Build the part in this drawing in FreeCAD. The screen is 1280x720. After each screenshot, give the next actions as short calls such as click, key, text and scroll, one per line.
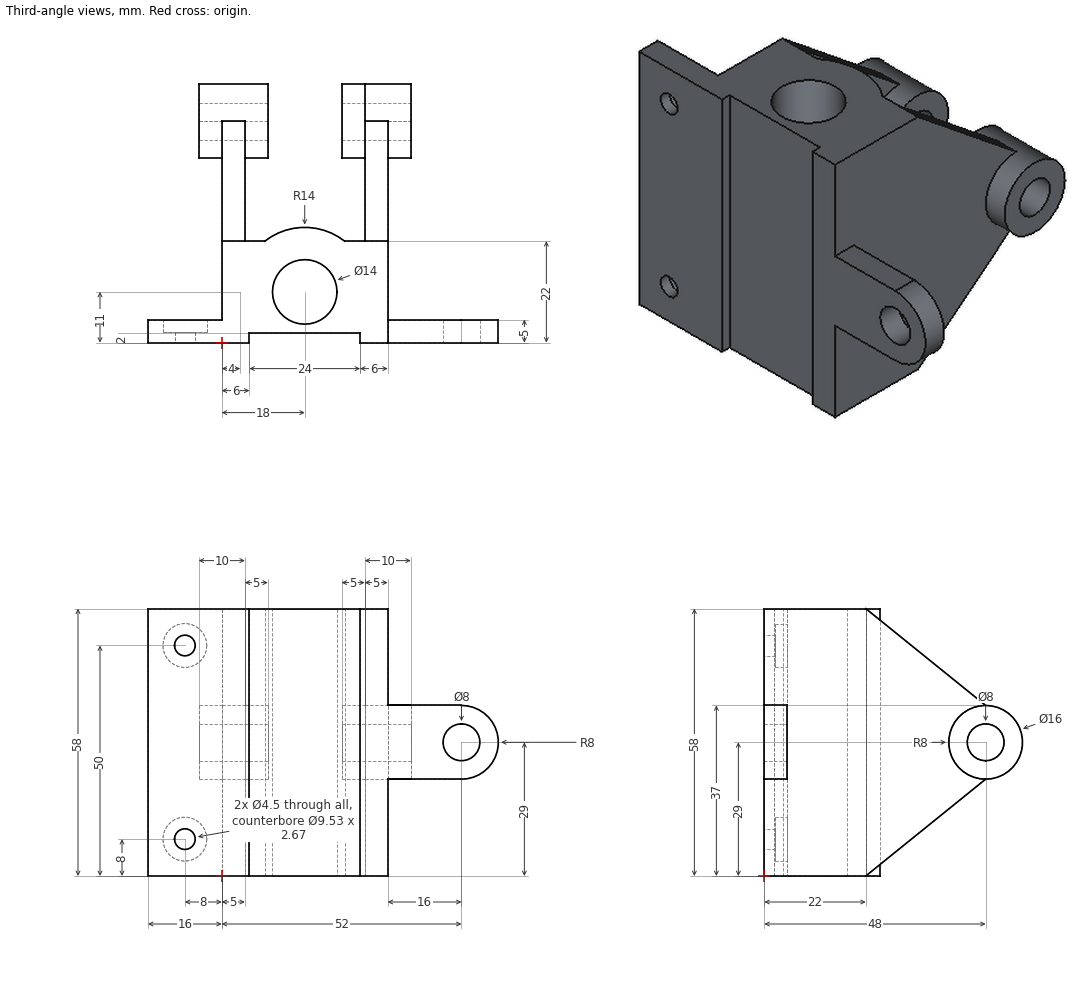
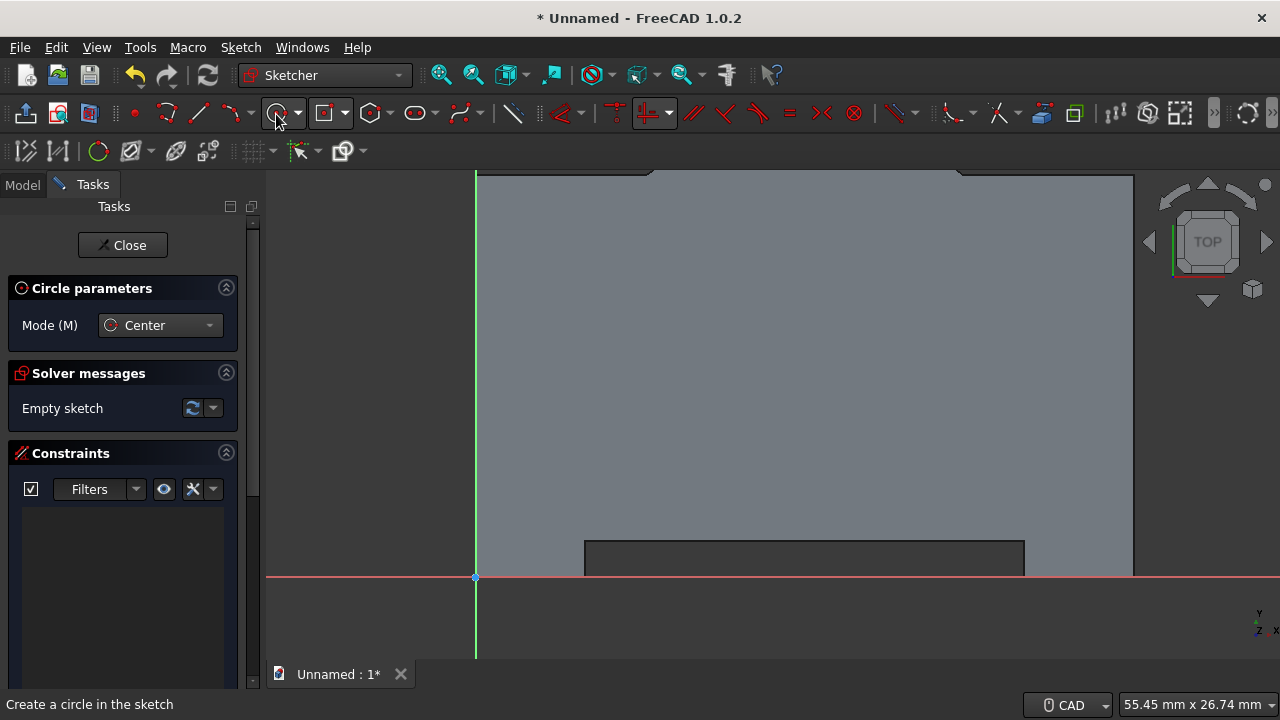
click(805, 376)
move(895, 286)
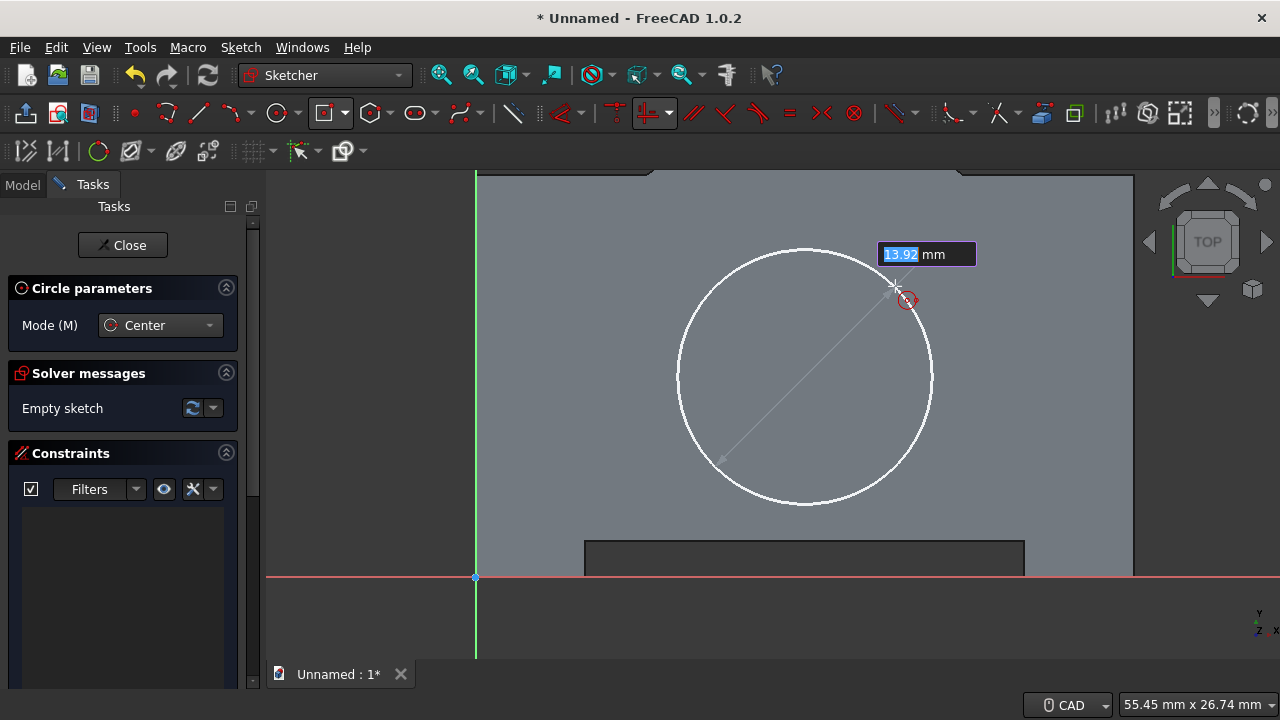
text(14)
key(Return)
key(Escape)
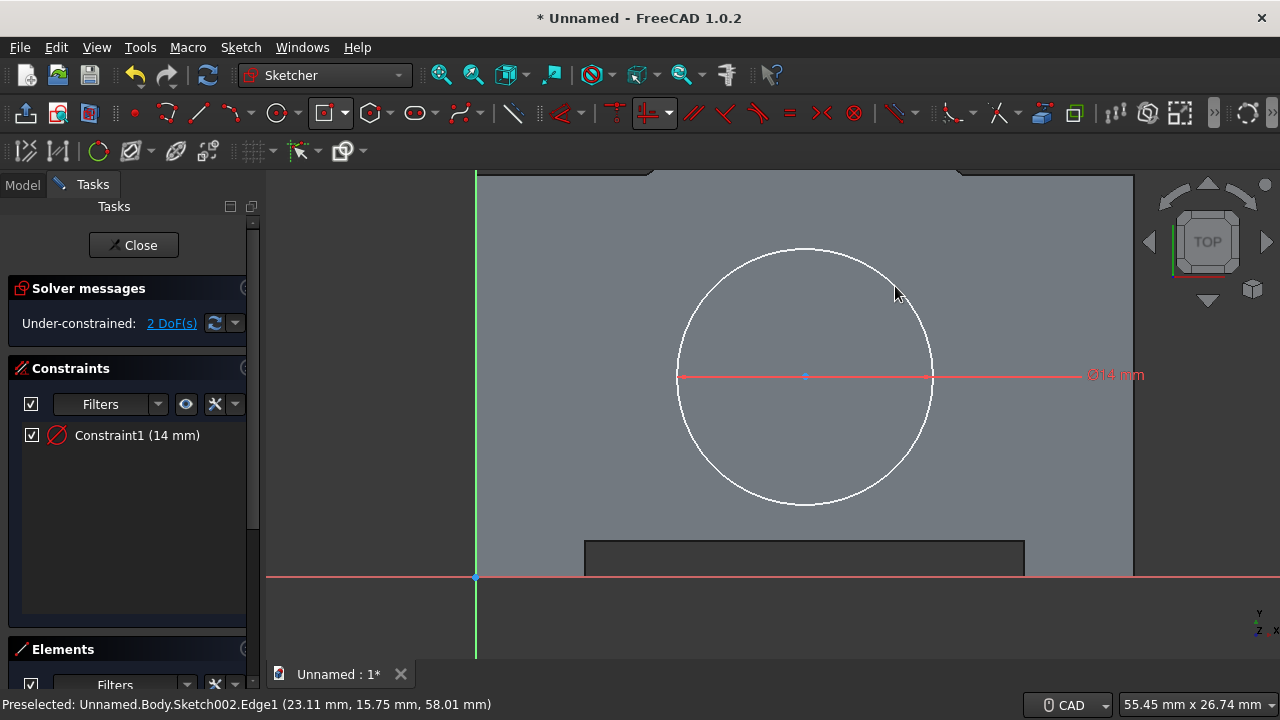
click(560, 114)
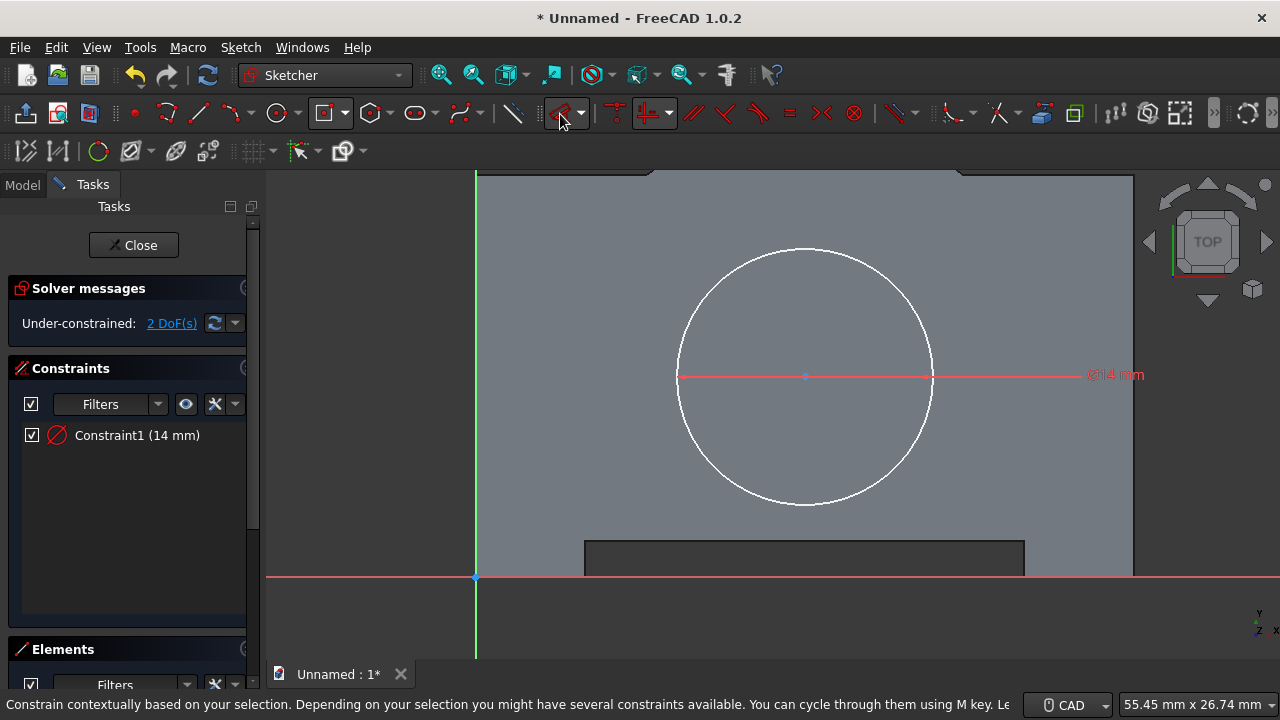
click(805, 377)
click(640, 611)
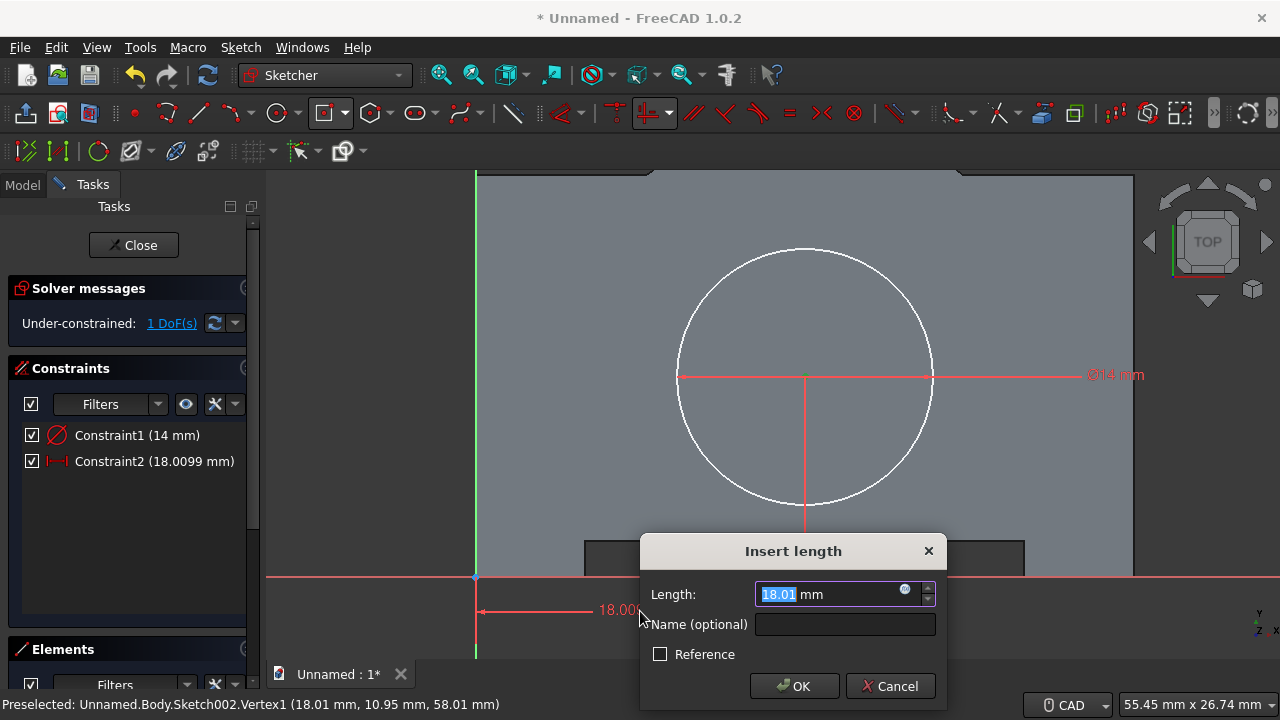
text(18)
key(Return)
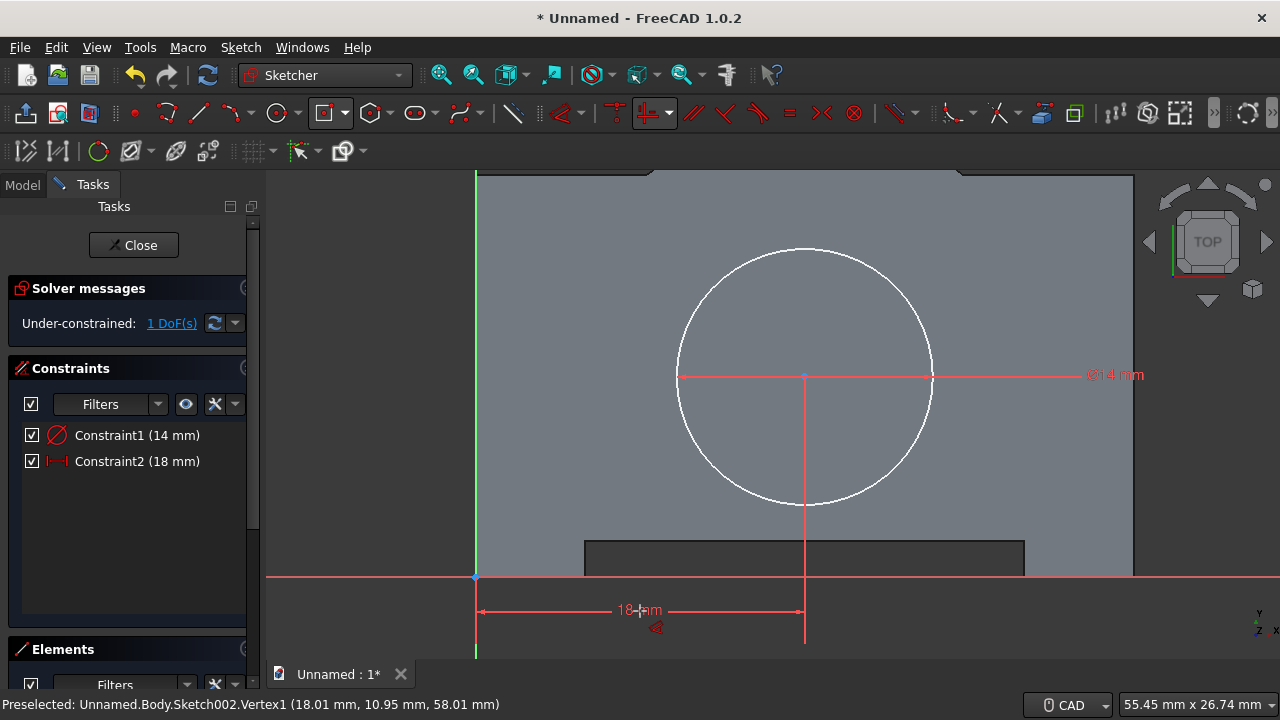
click(805, 377)
click(442, 477)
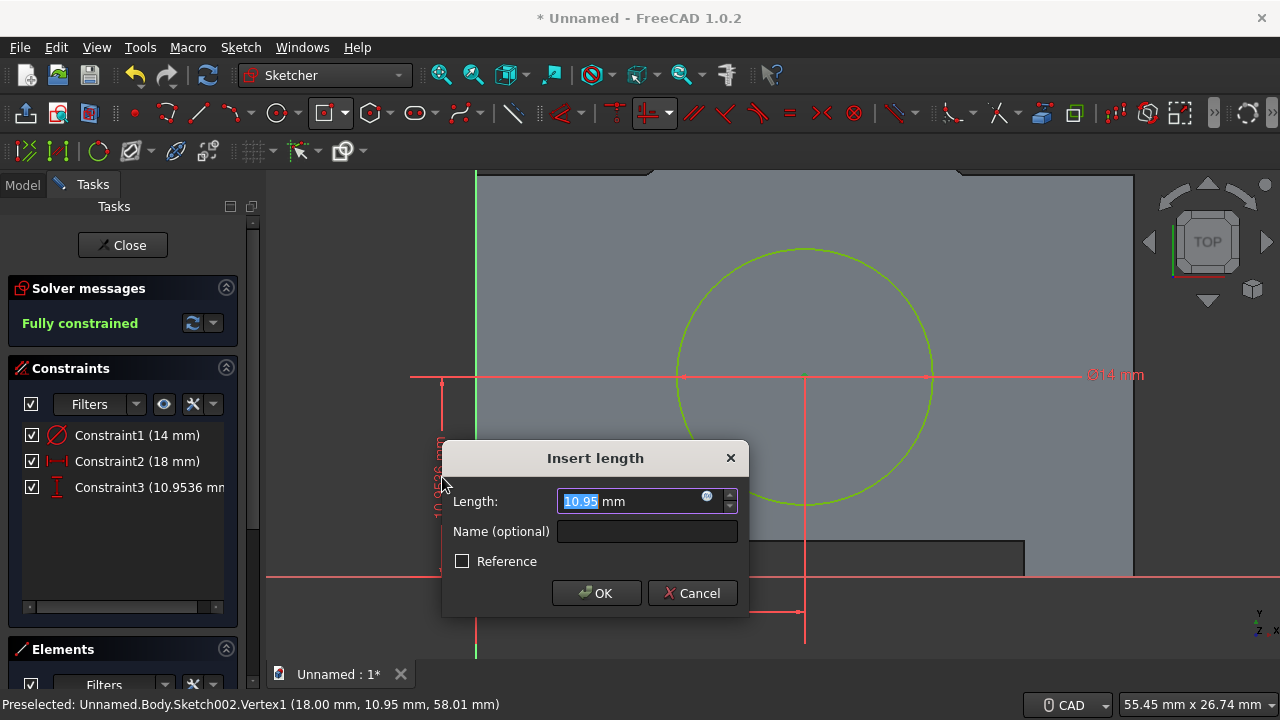
text(11)
key(Return)
key(Escape)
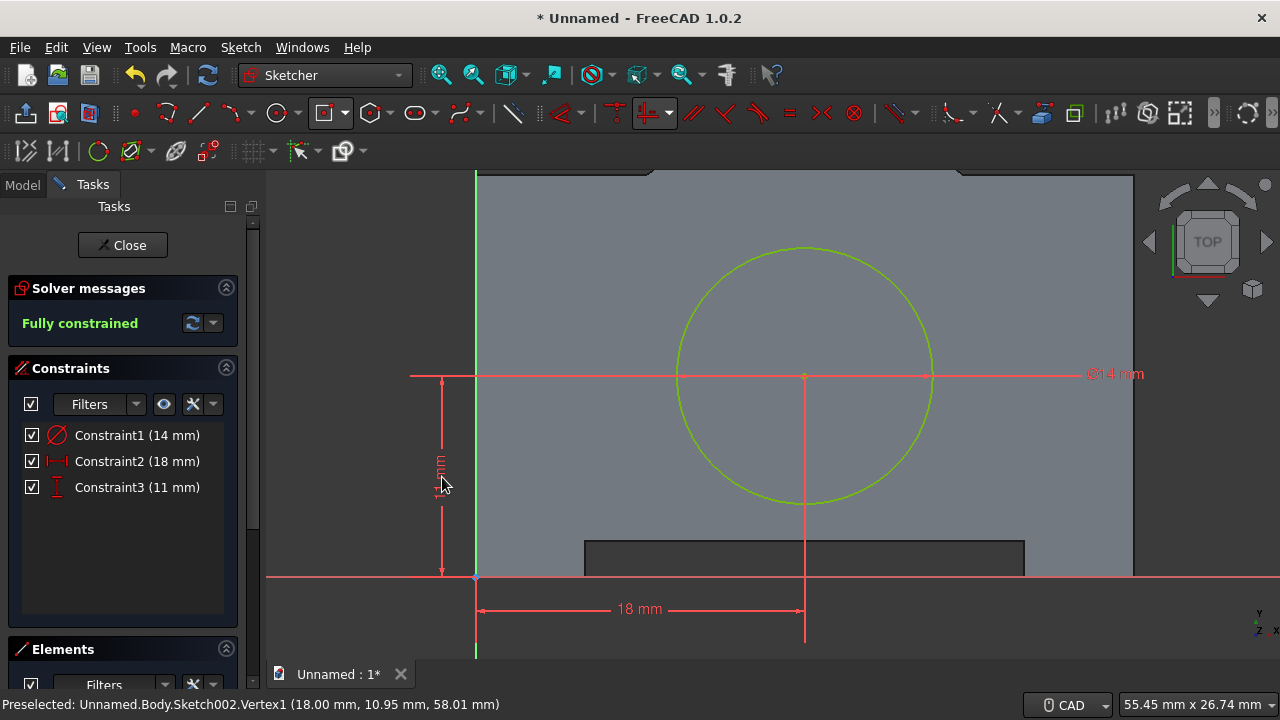
click(123, 245)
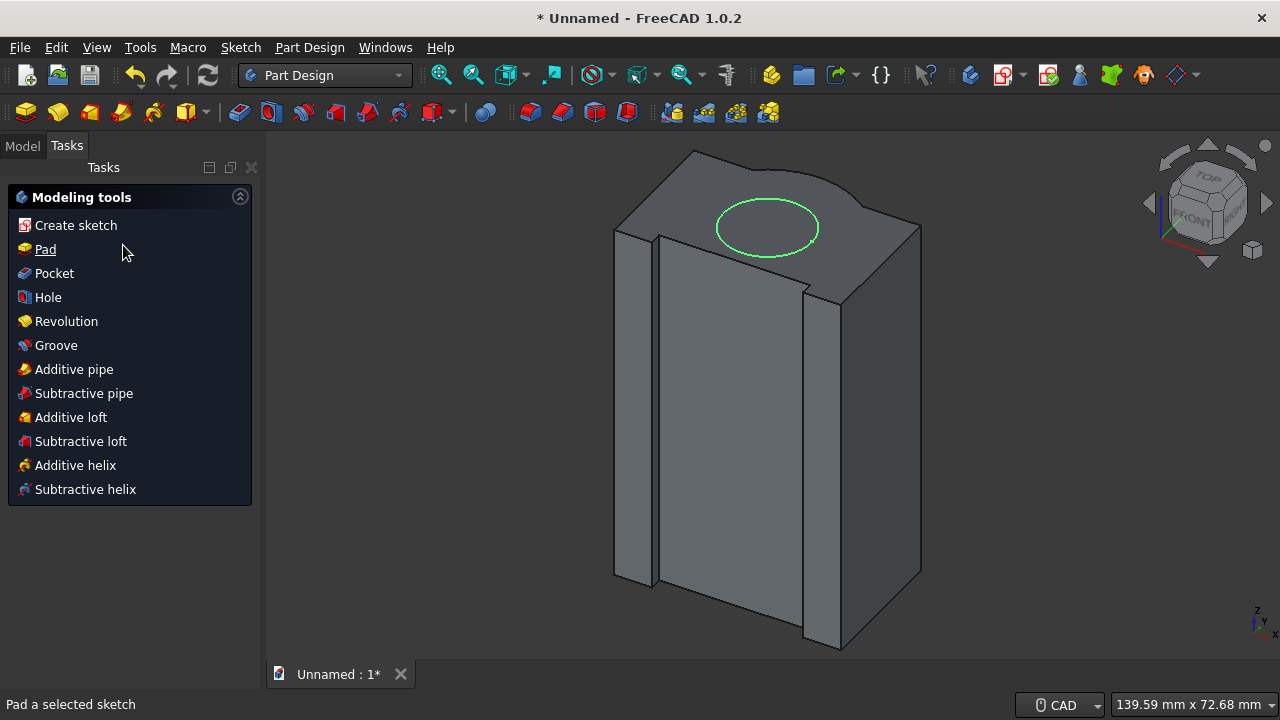
click(240, 112)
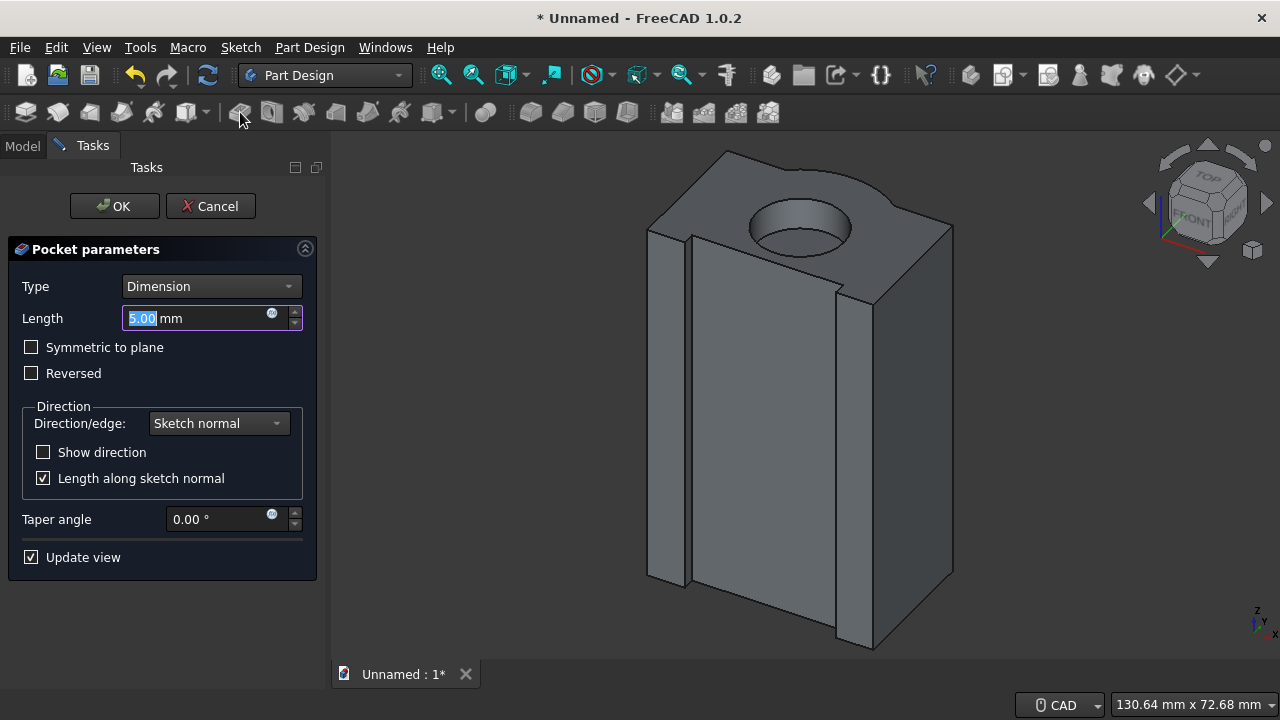
click(212, 286)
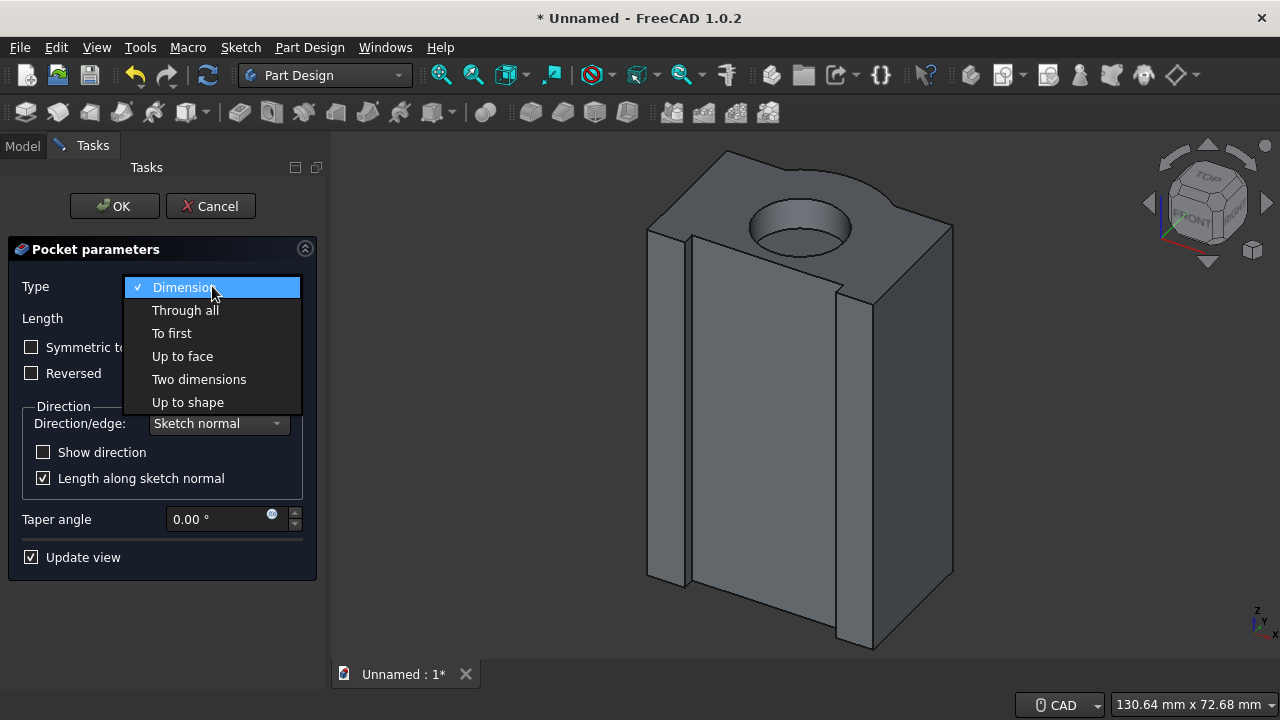
click(212, 310)